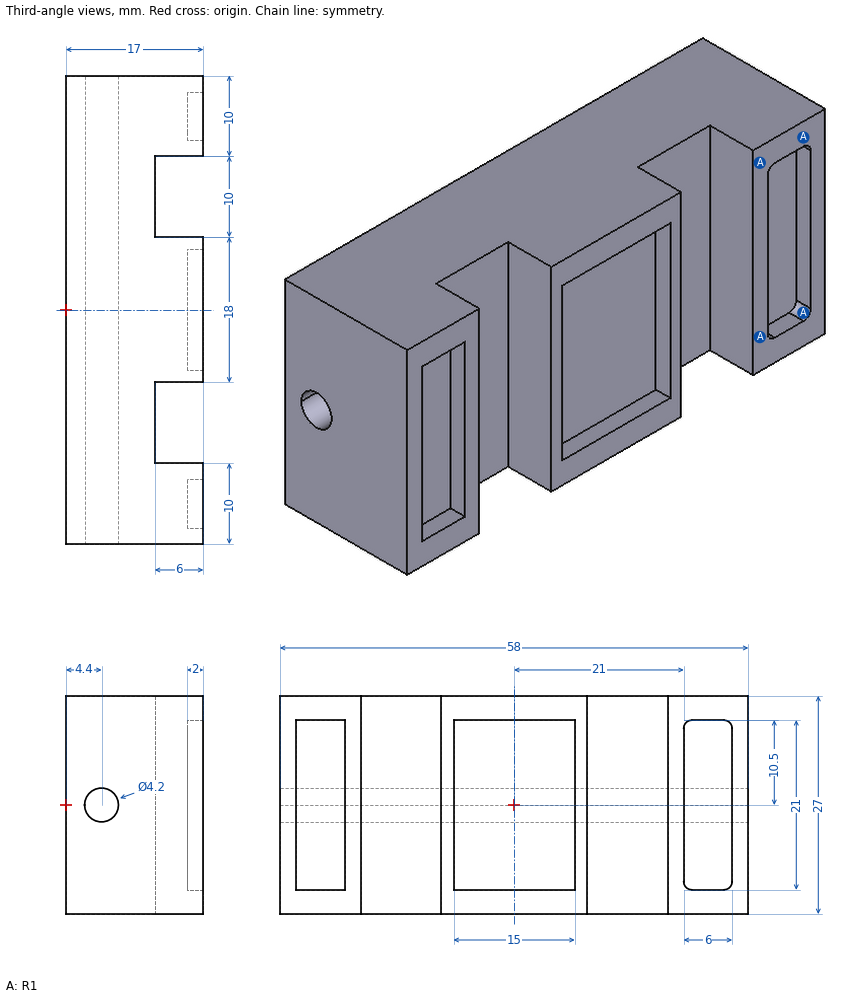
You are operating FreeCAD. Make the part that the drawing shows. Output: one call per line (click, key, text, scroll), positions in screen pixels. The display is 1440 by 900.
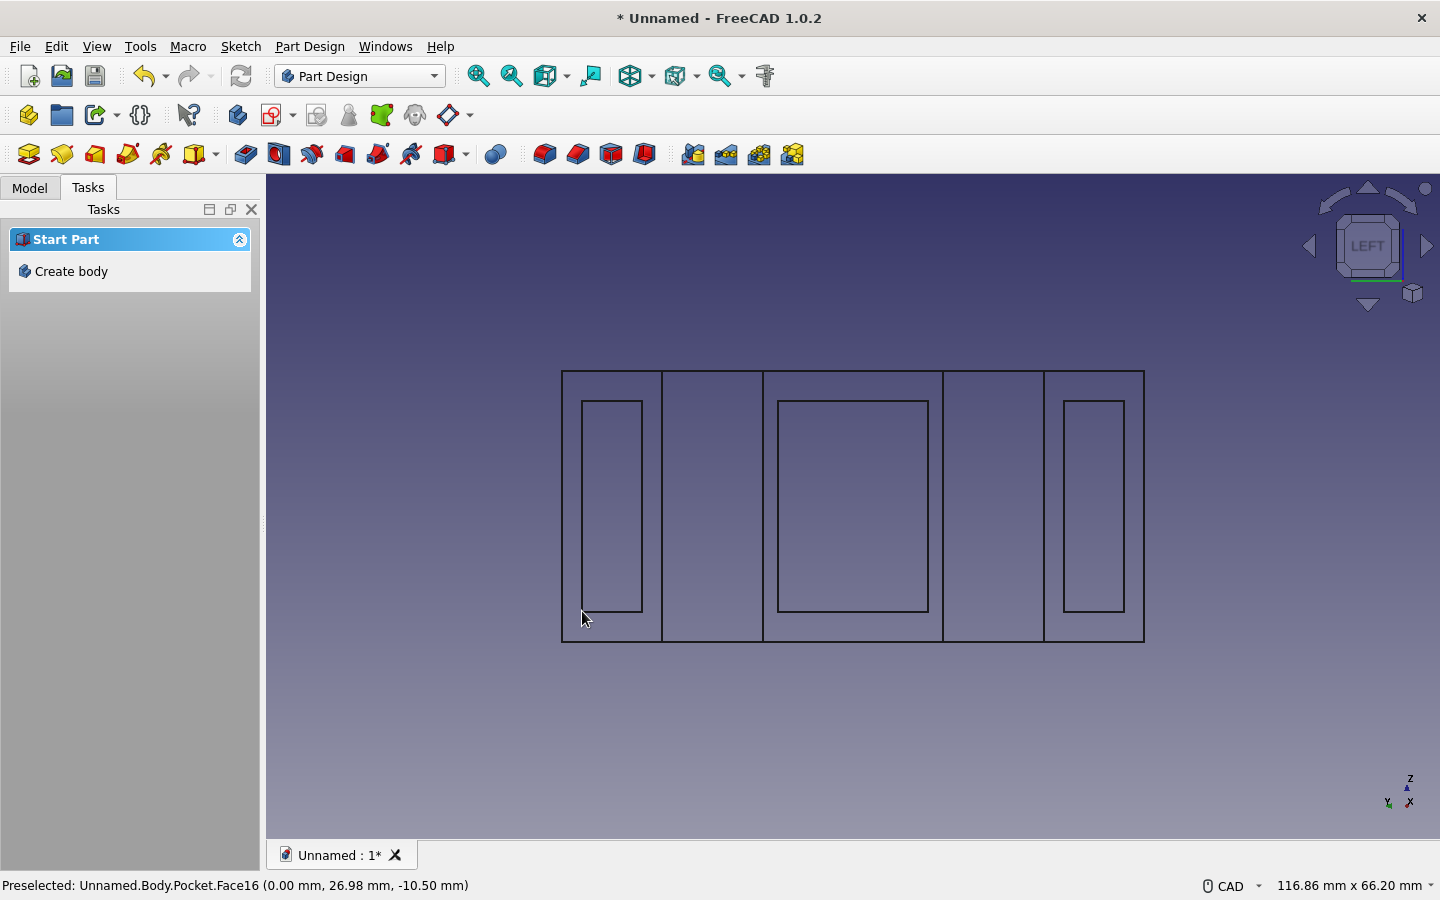
key(0)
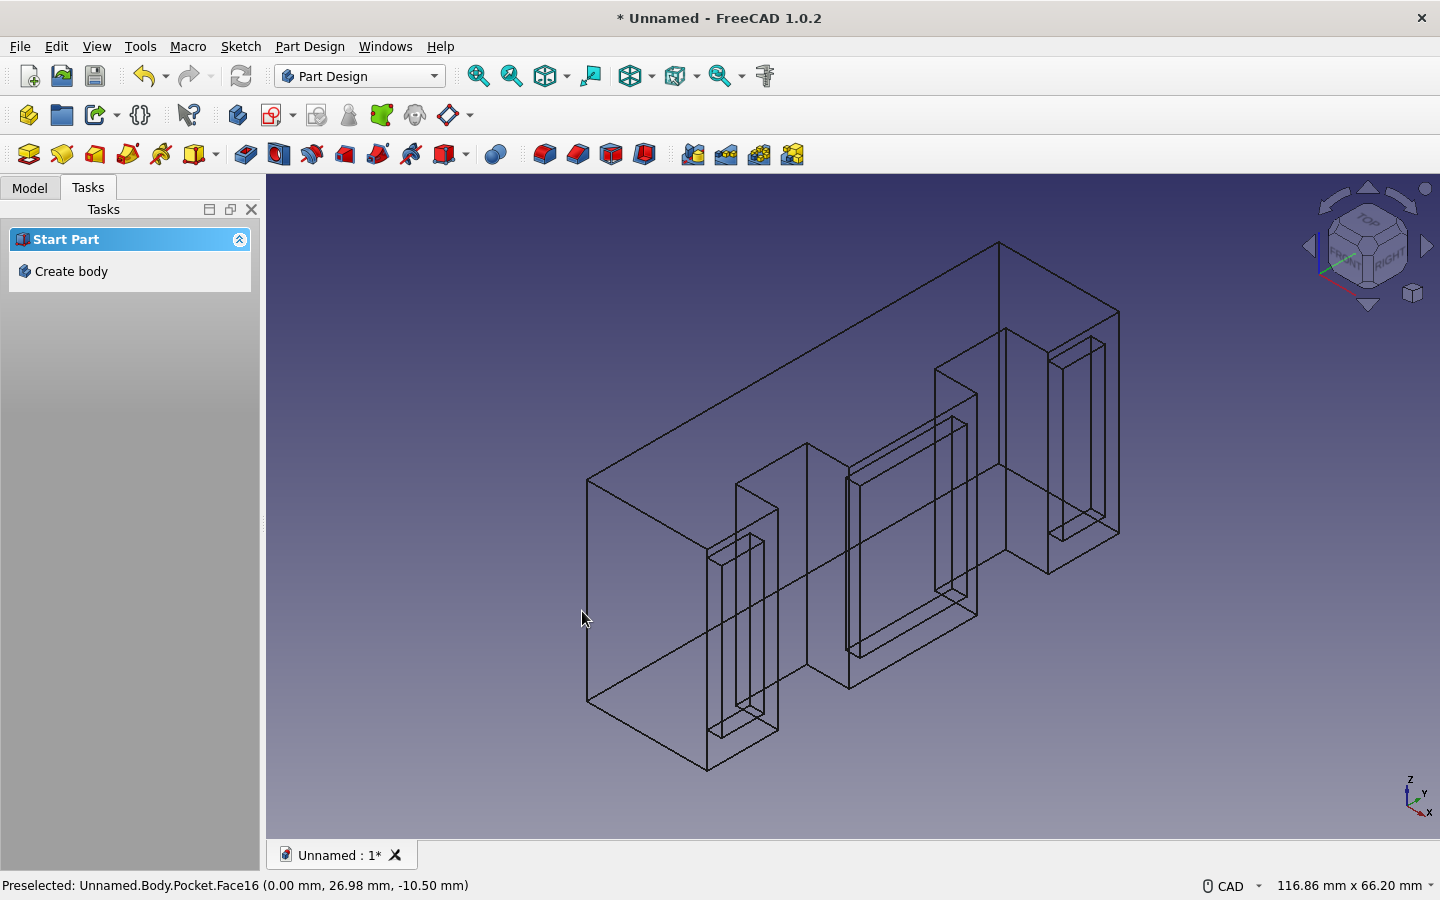
click(1098, 512)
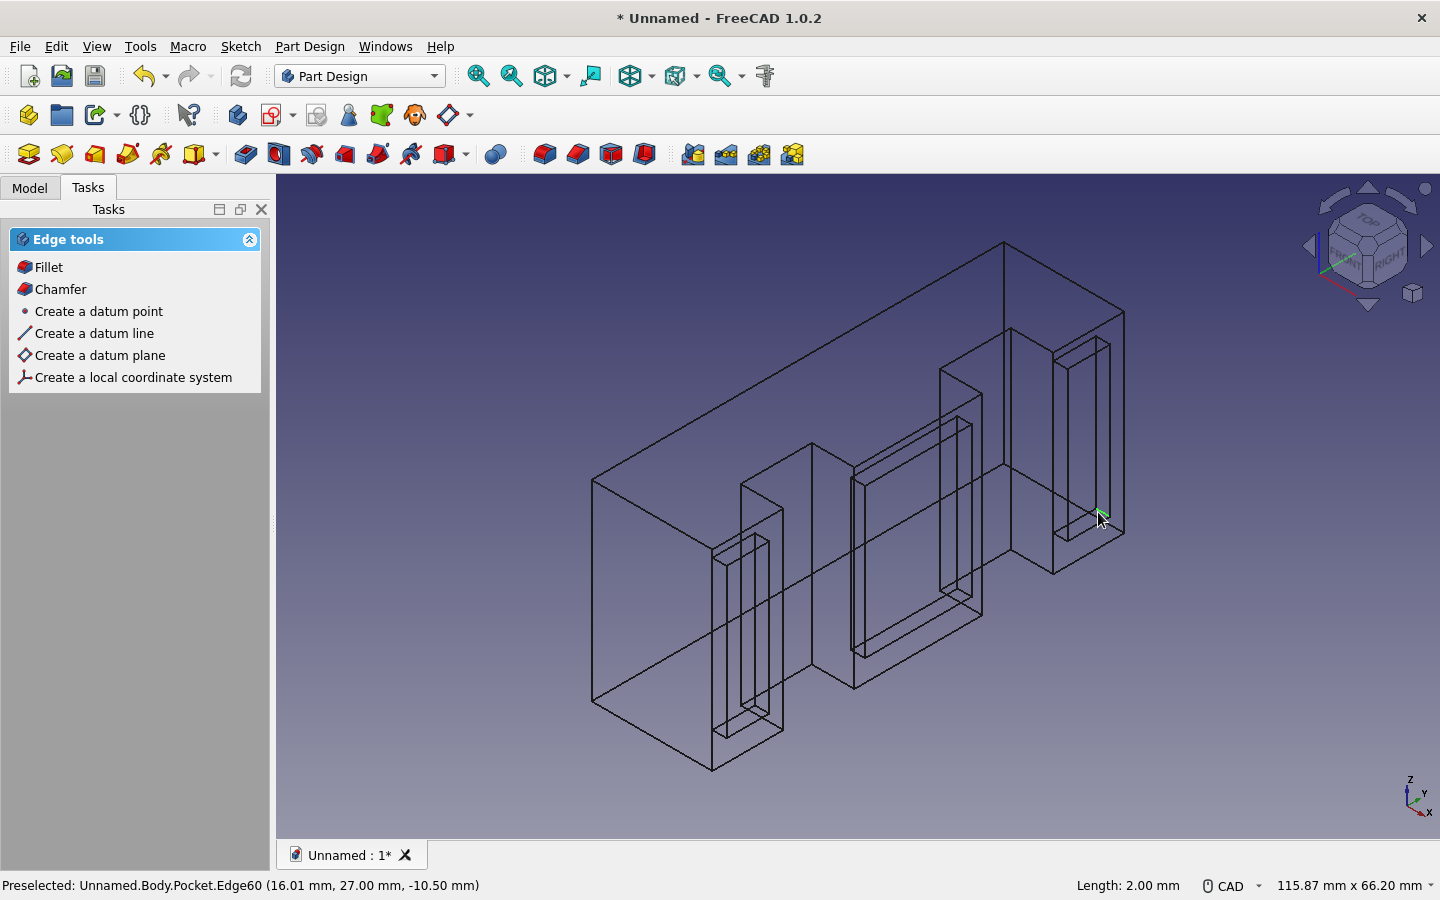
click(1060, 536, ctrl)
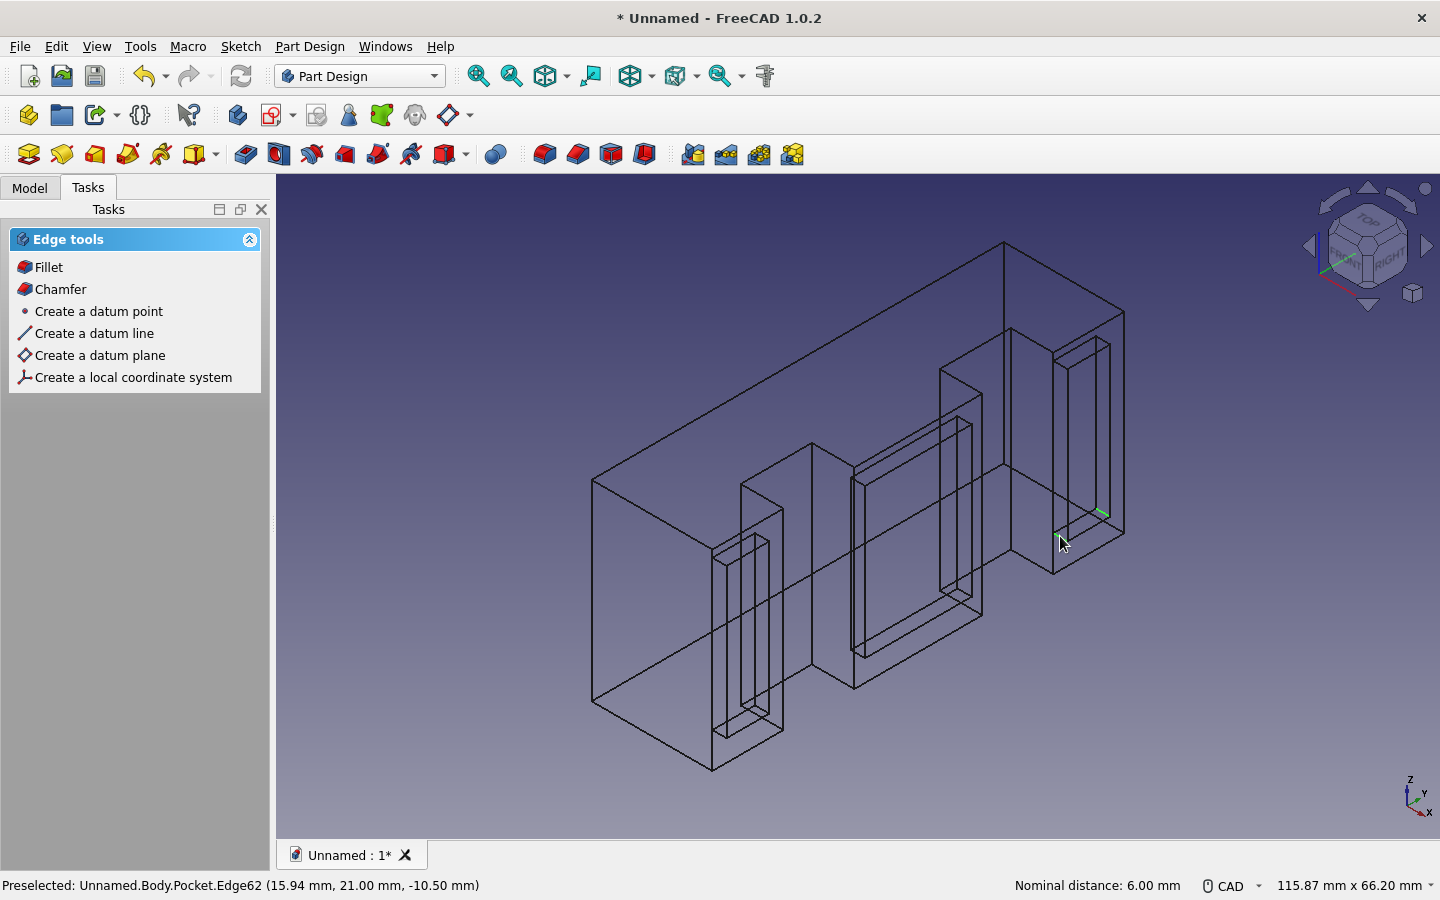
click(1060, 364, ctrl)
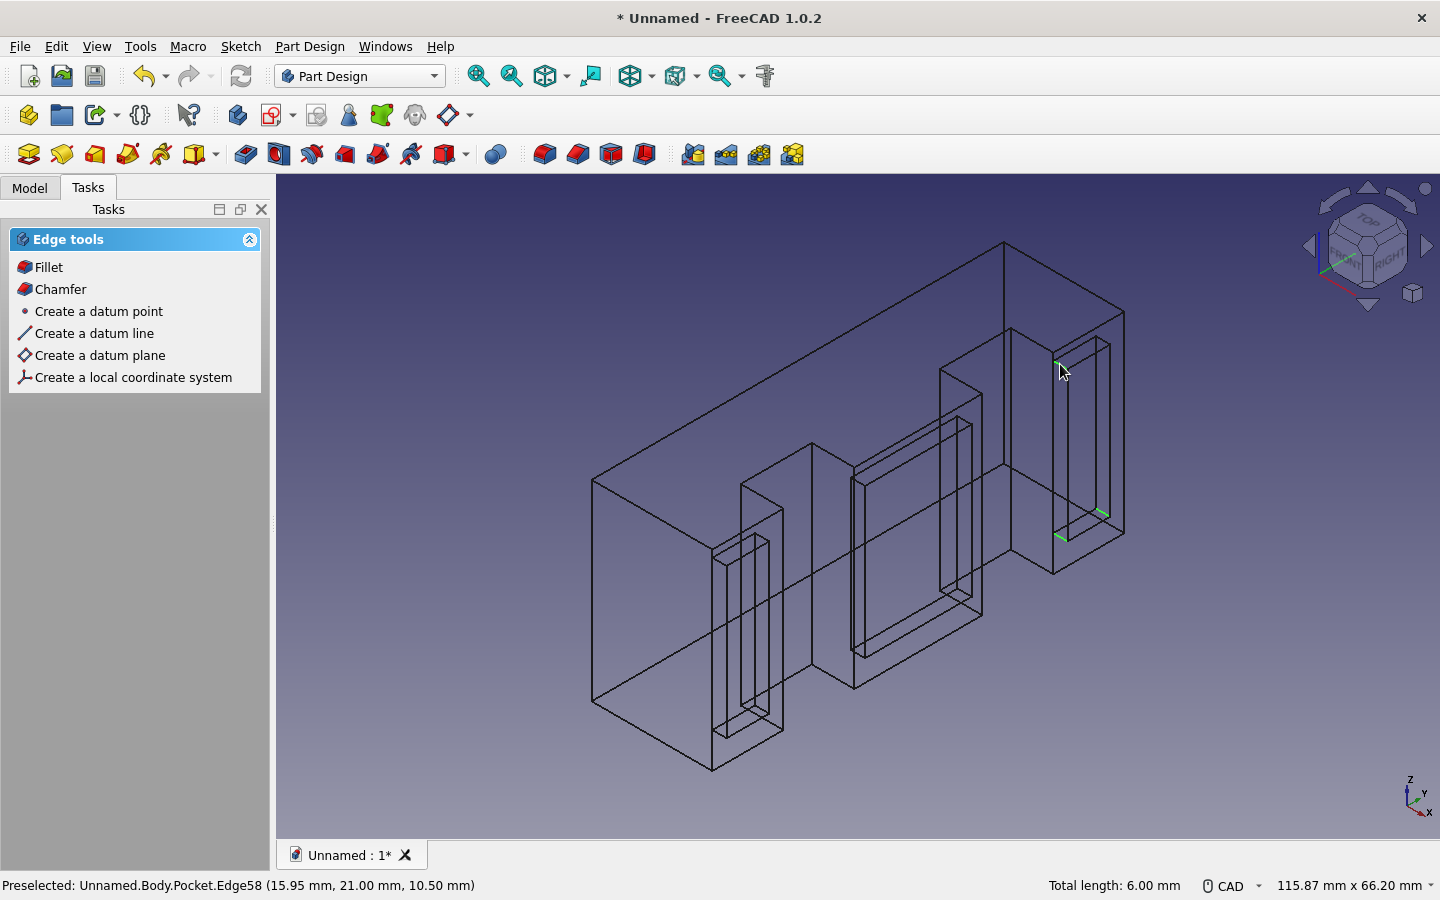
click(1103, 339, ctrl)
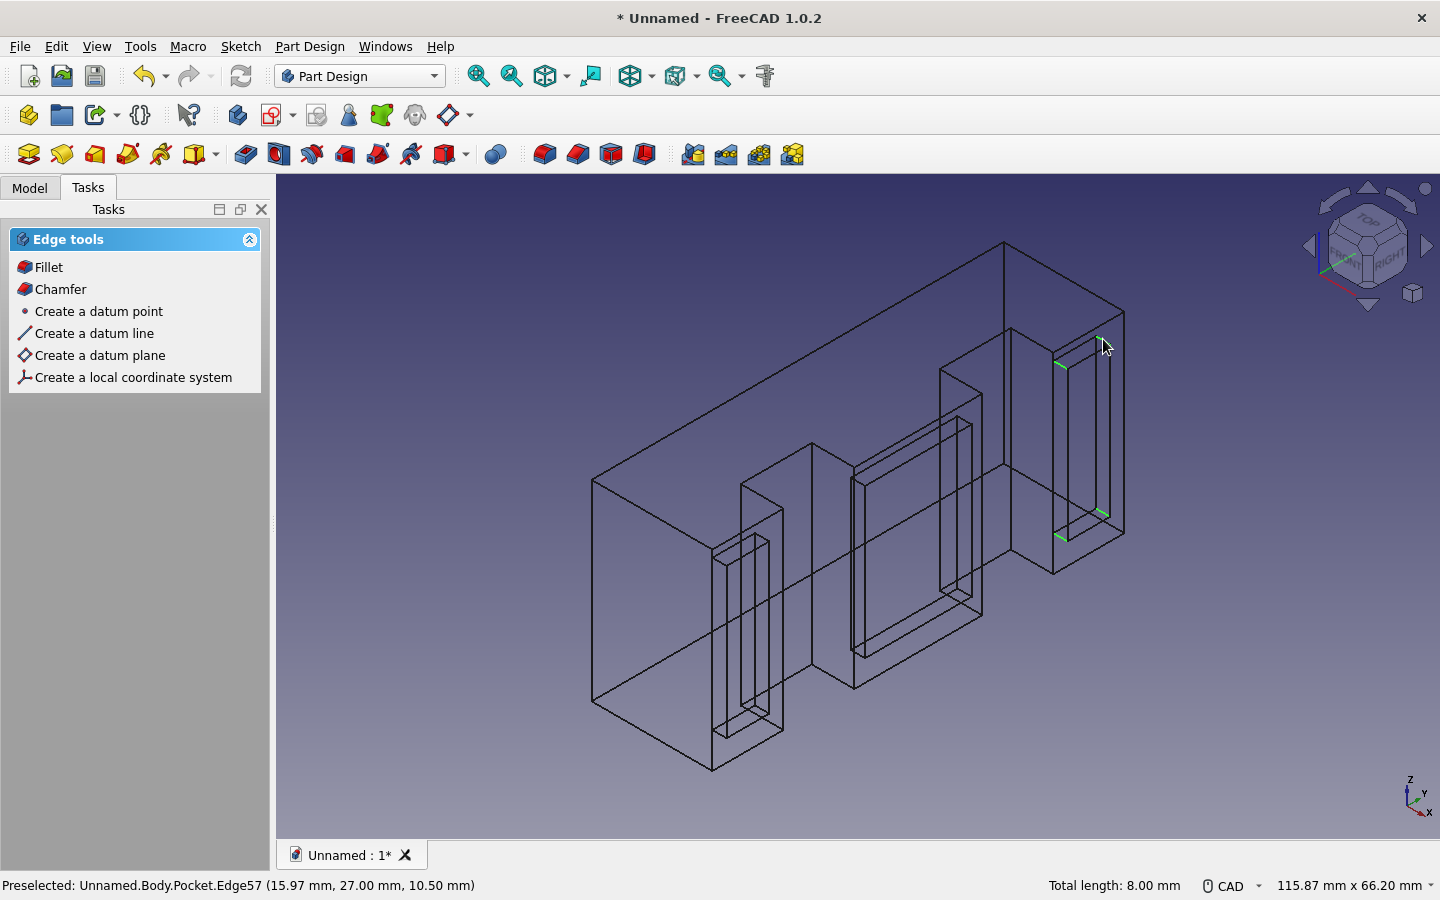
key(v)
key(1)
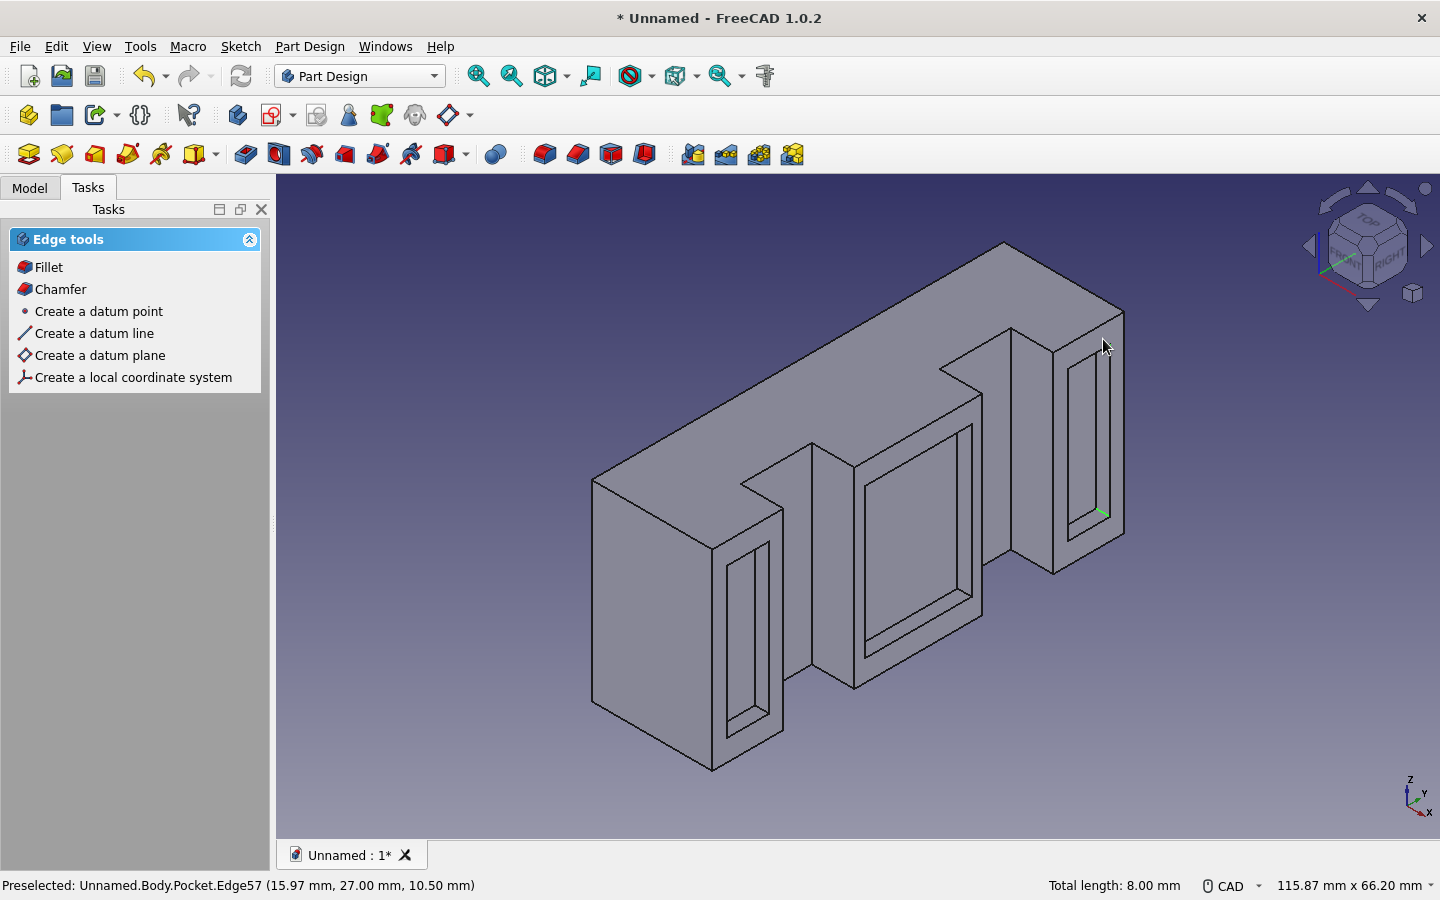
click(545, 154)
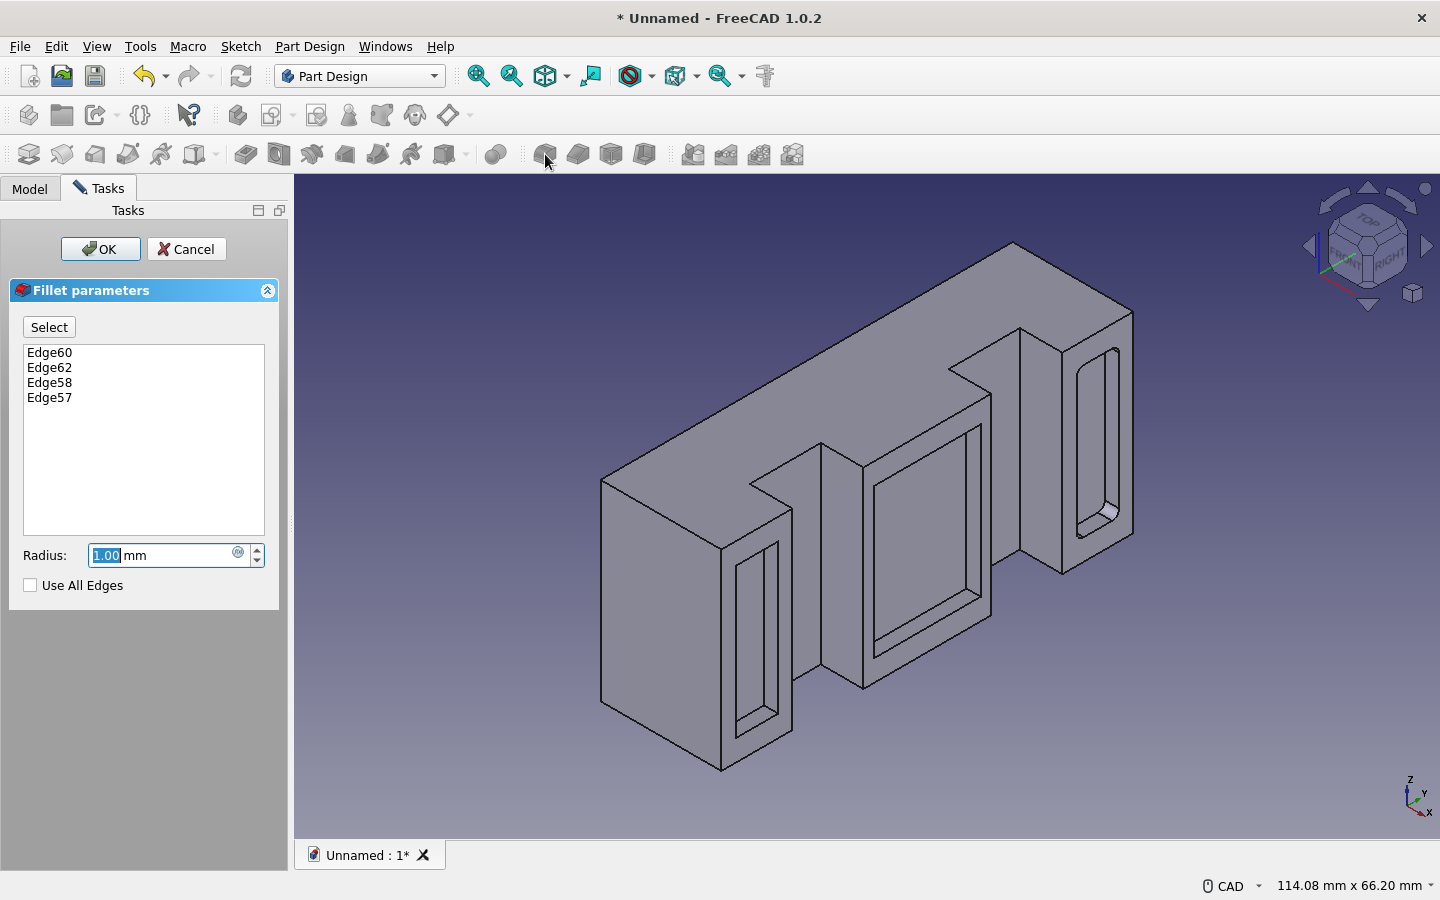
text(1)
key(Tab)